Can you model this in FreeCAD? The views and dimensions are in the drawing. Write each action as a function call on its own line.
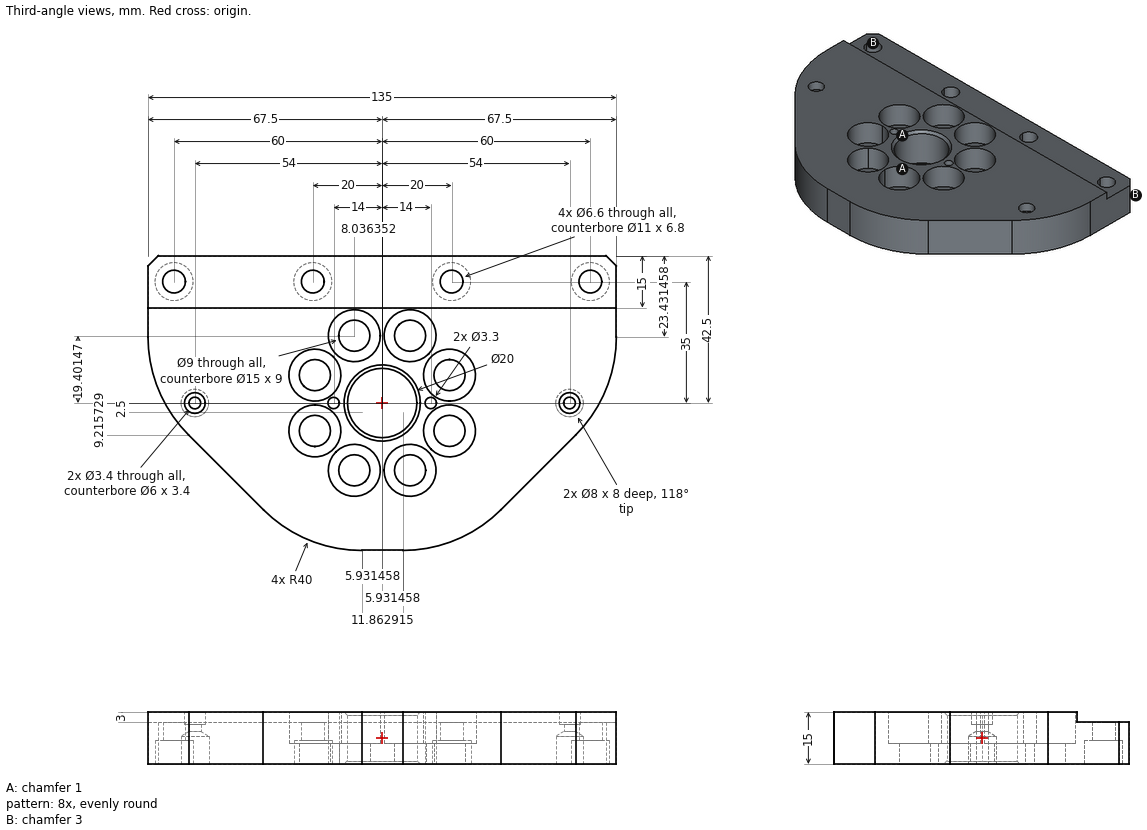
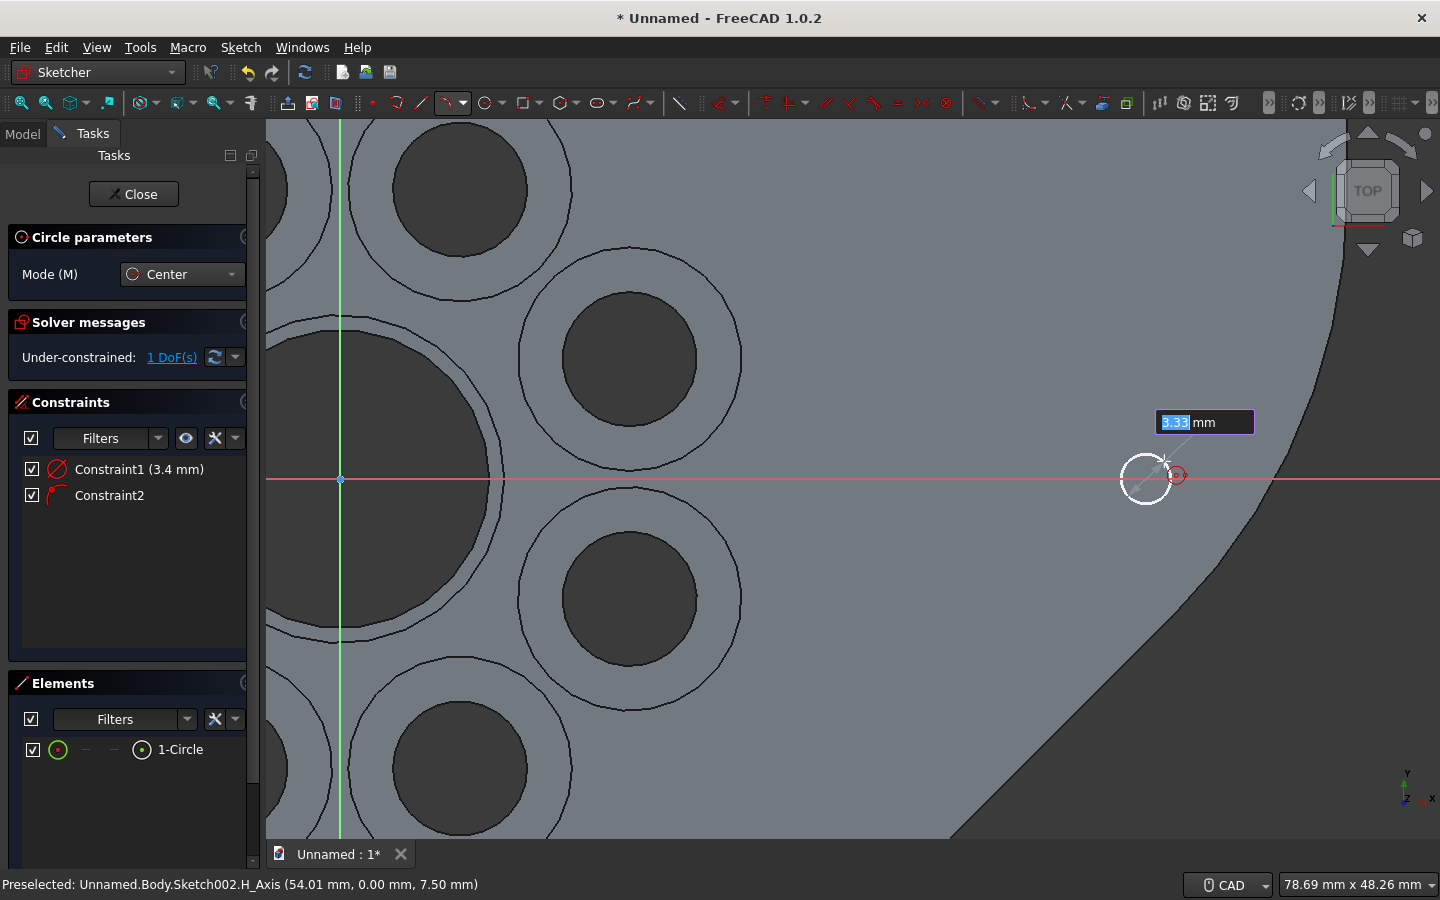
text(3.4)
key(Return)
key(Escape)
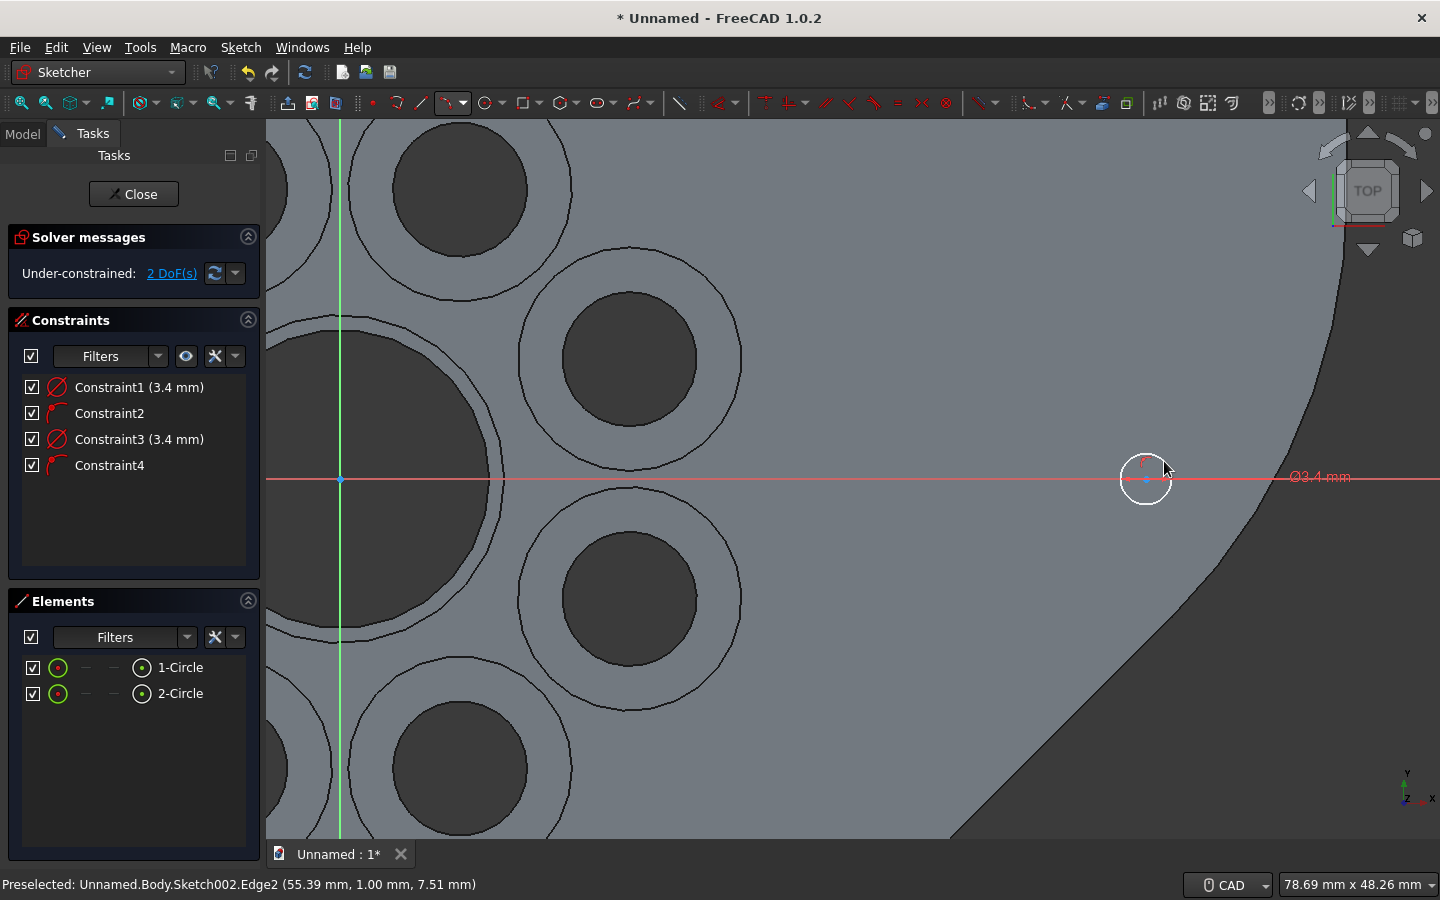
click(718, 104)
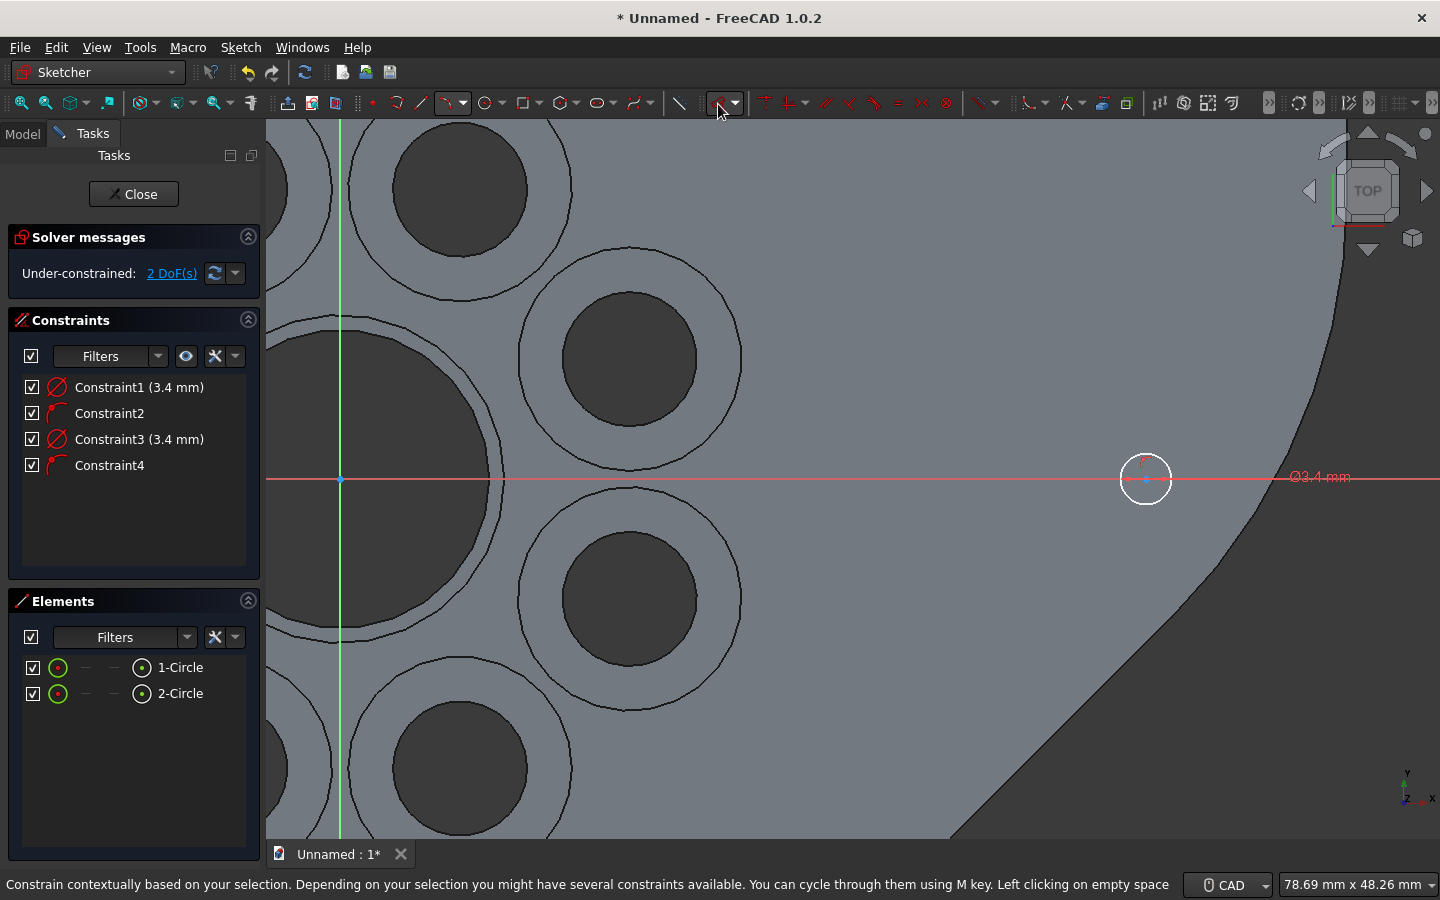
scroll(1147, 479, down, 4)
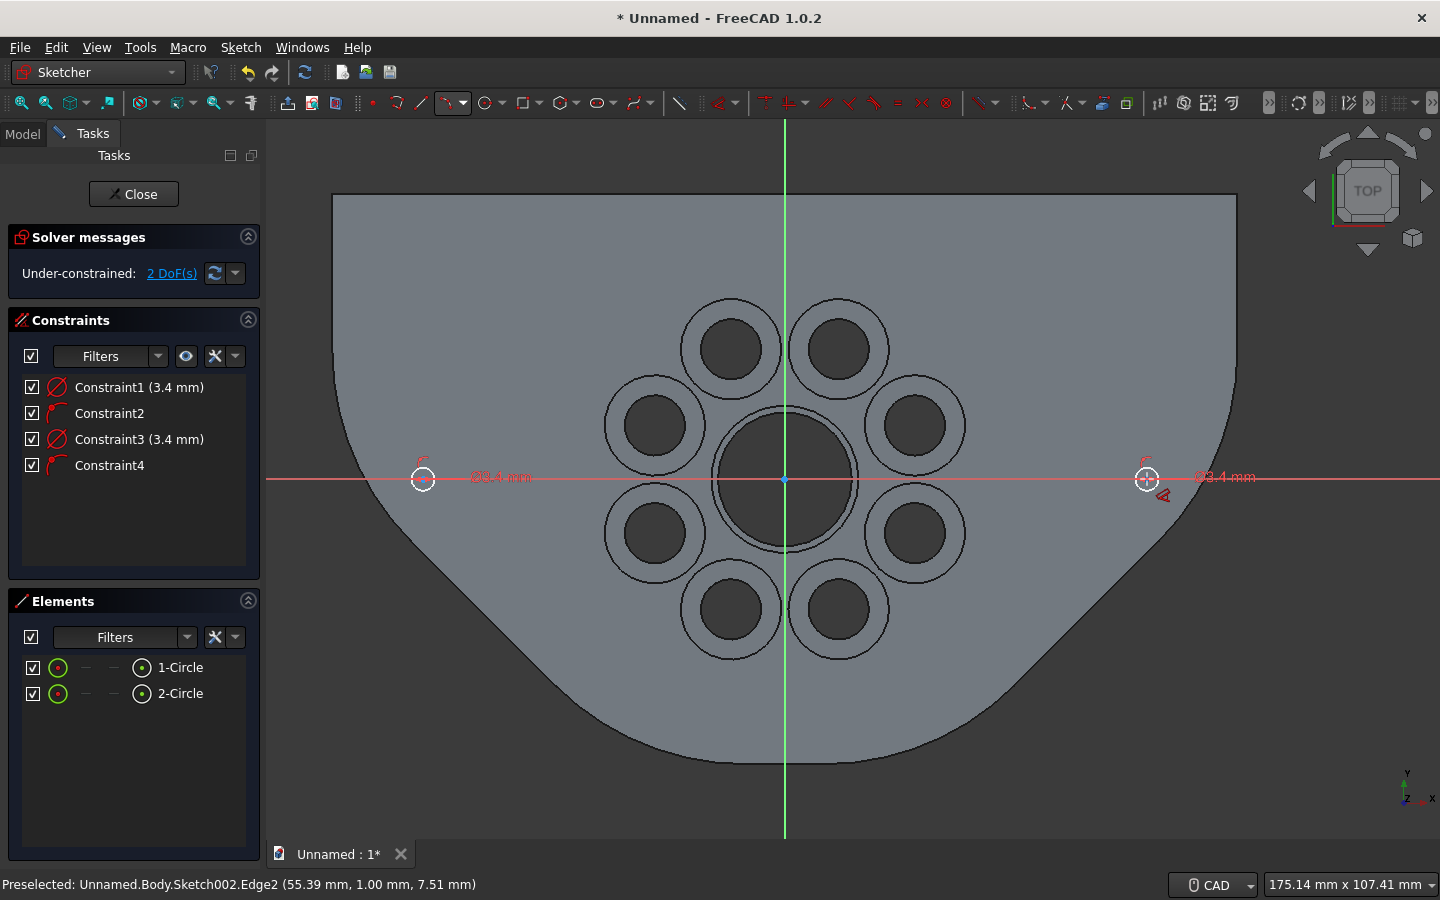
click(423, 479)
click(604, 513)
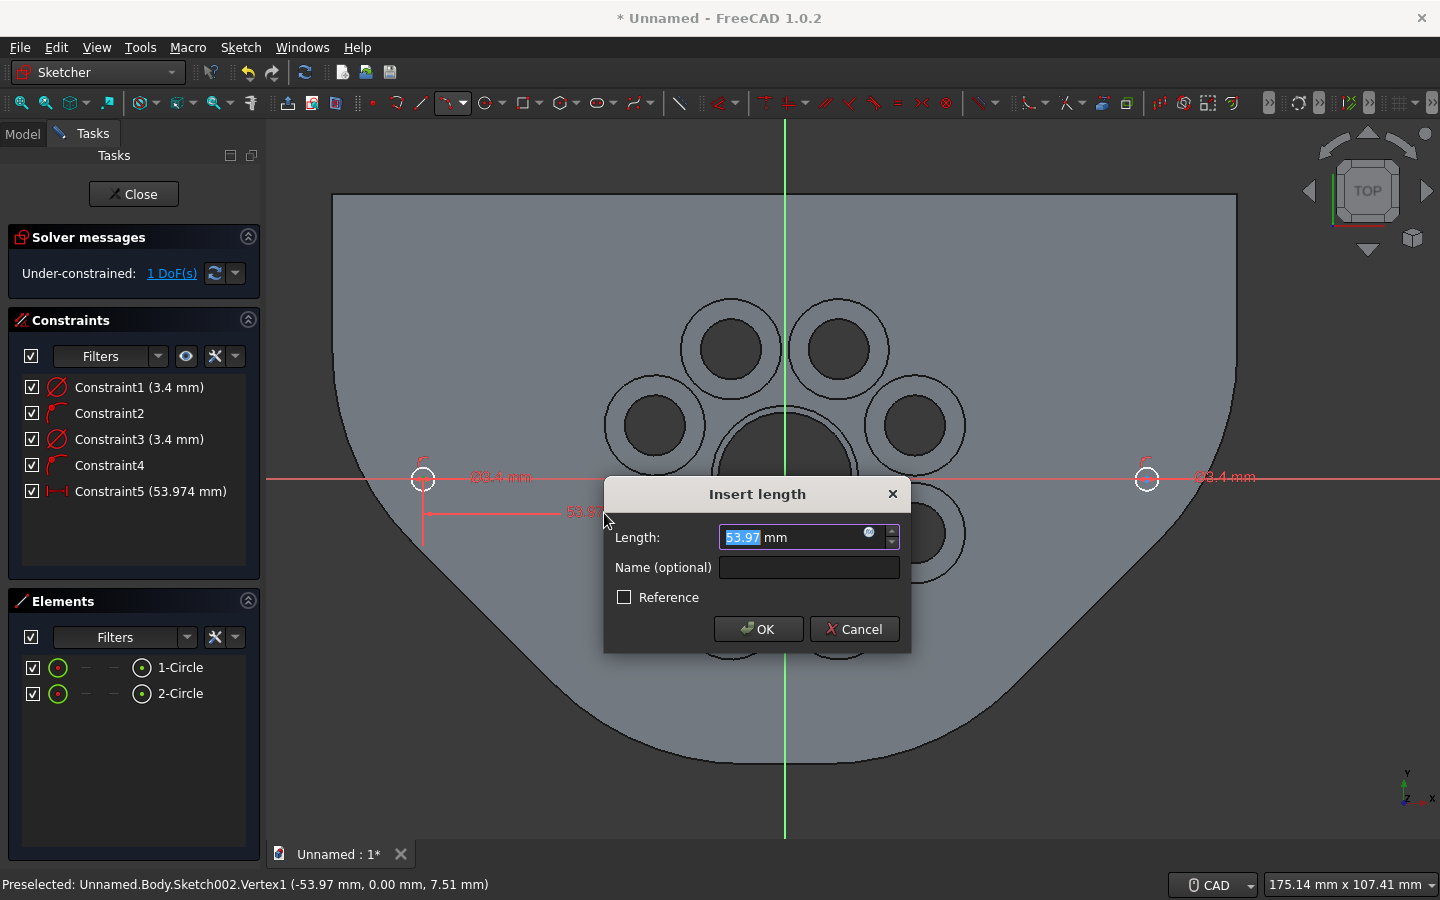
text(54)
key(Return)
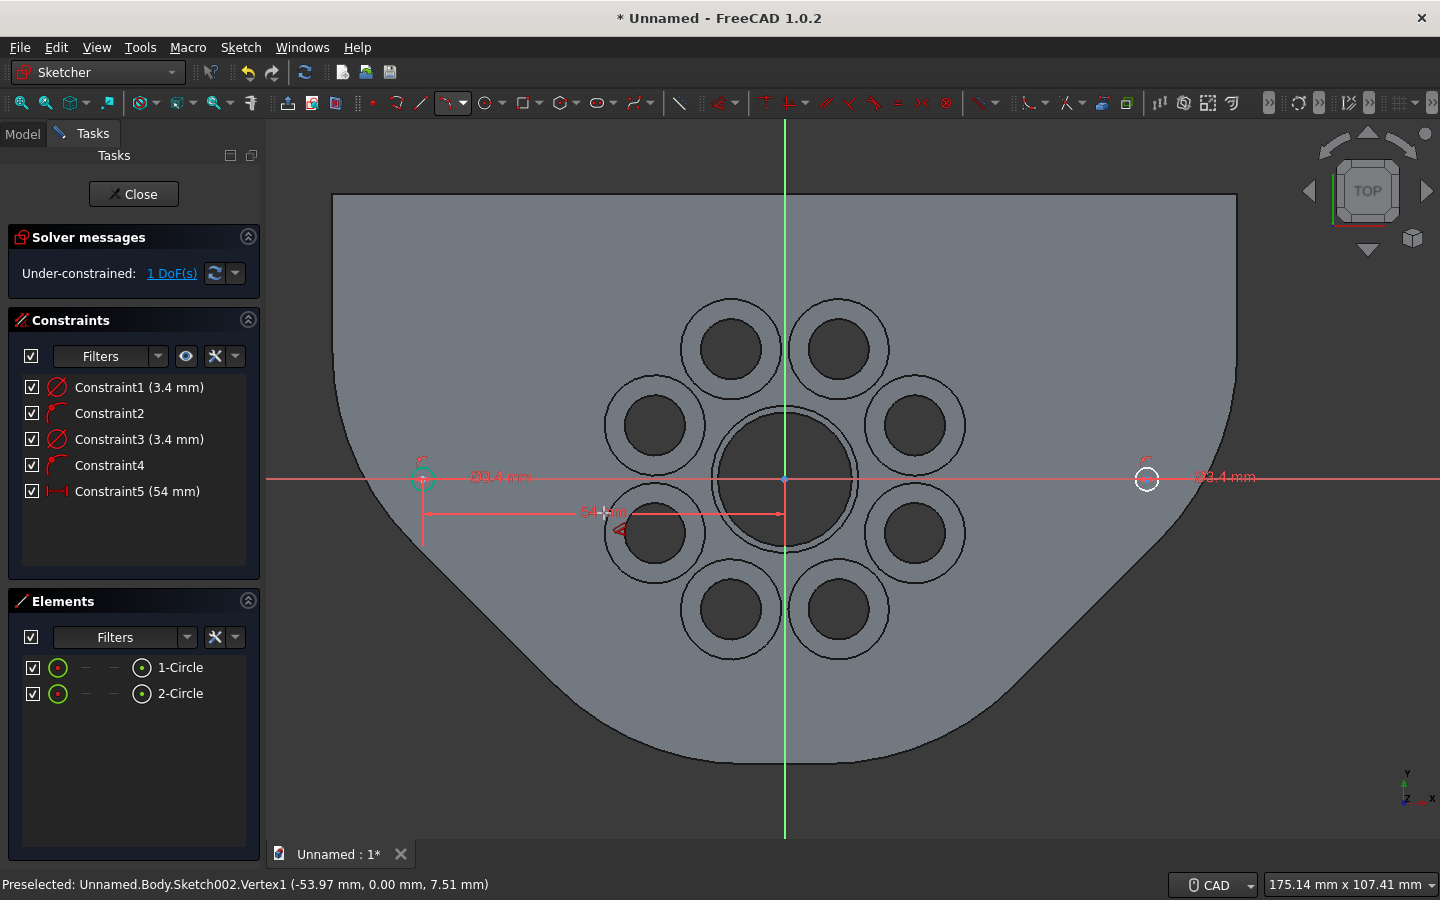
click(1147, 479)
click(966, 513)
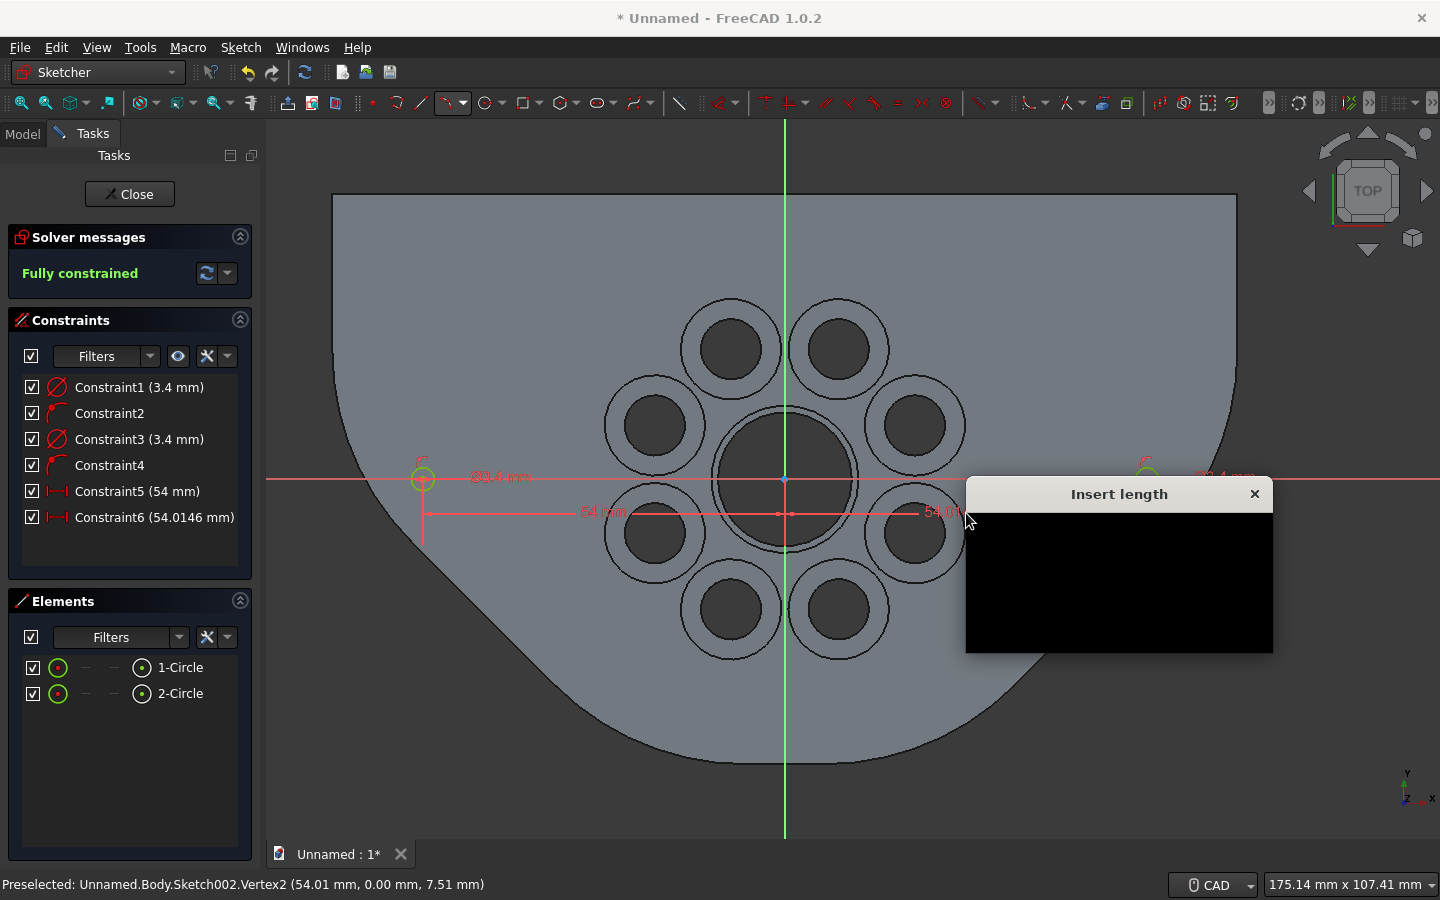
text(54)
key(Return)
key(Escape)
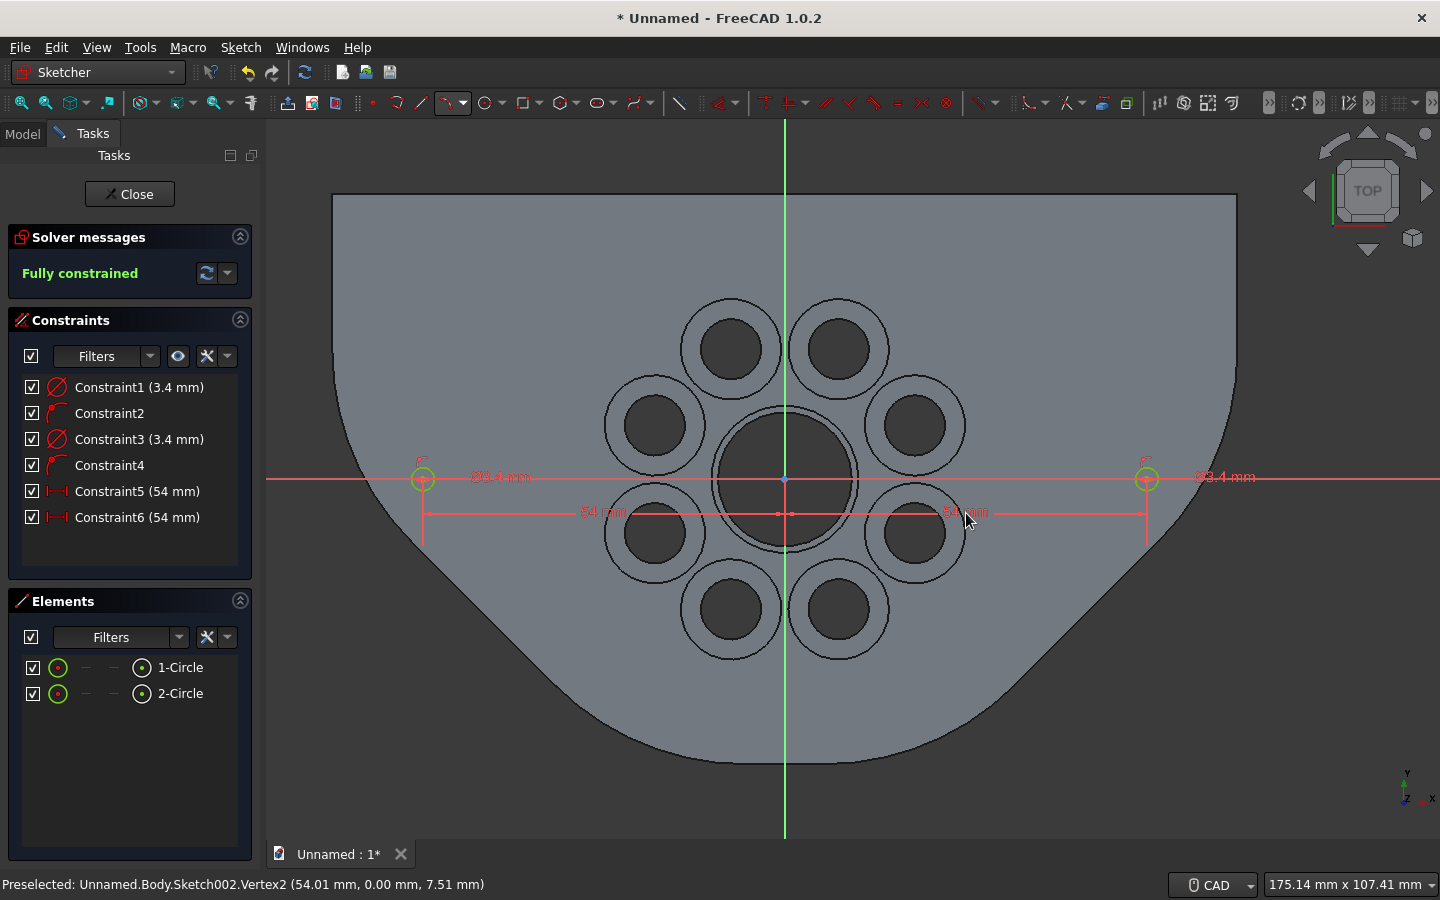
click(130, 194)